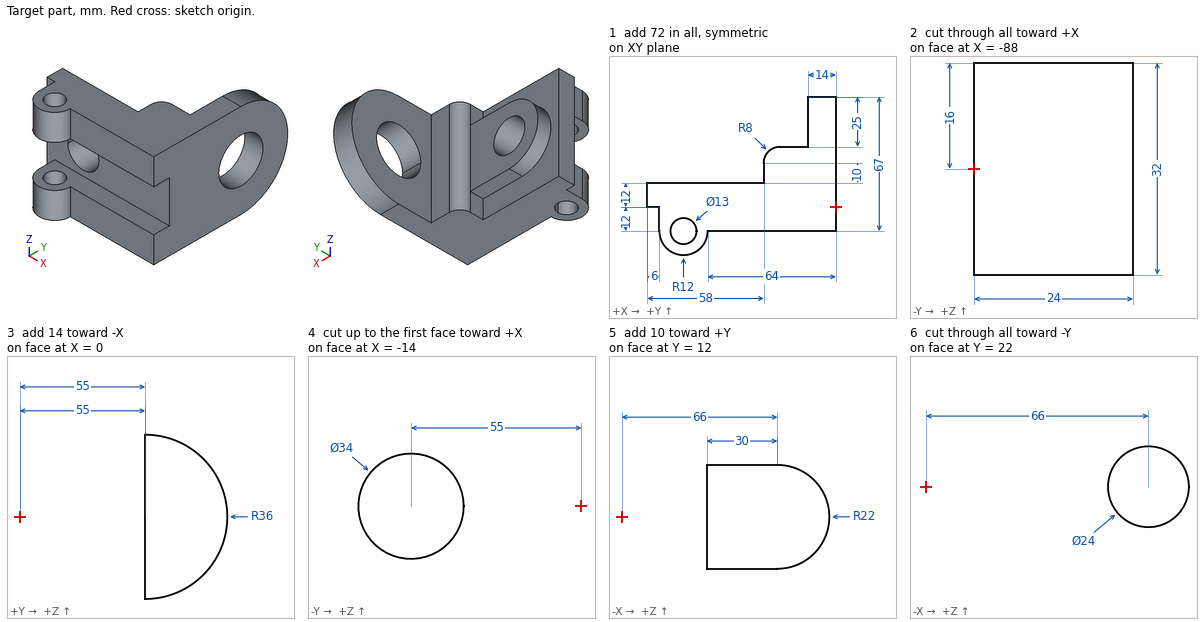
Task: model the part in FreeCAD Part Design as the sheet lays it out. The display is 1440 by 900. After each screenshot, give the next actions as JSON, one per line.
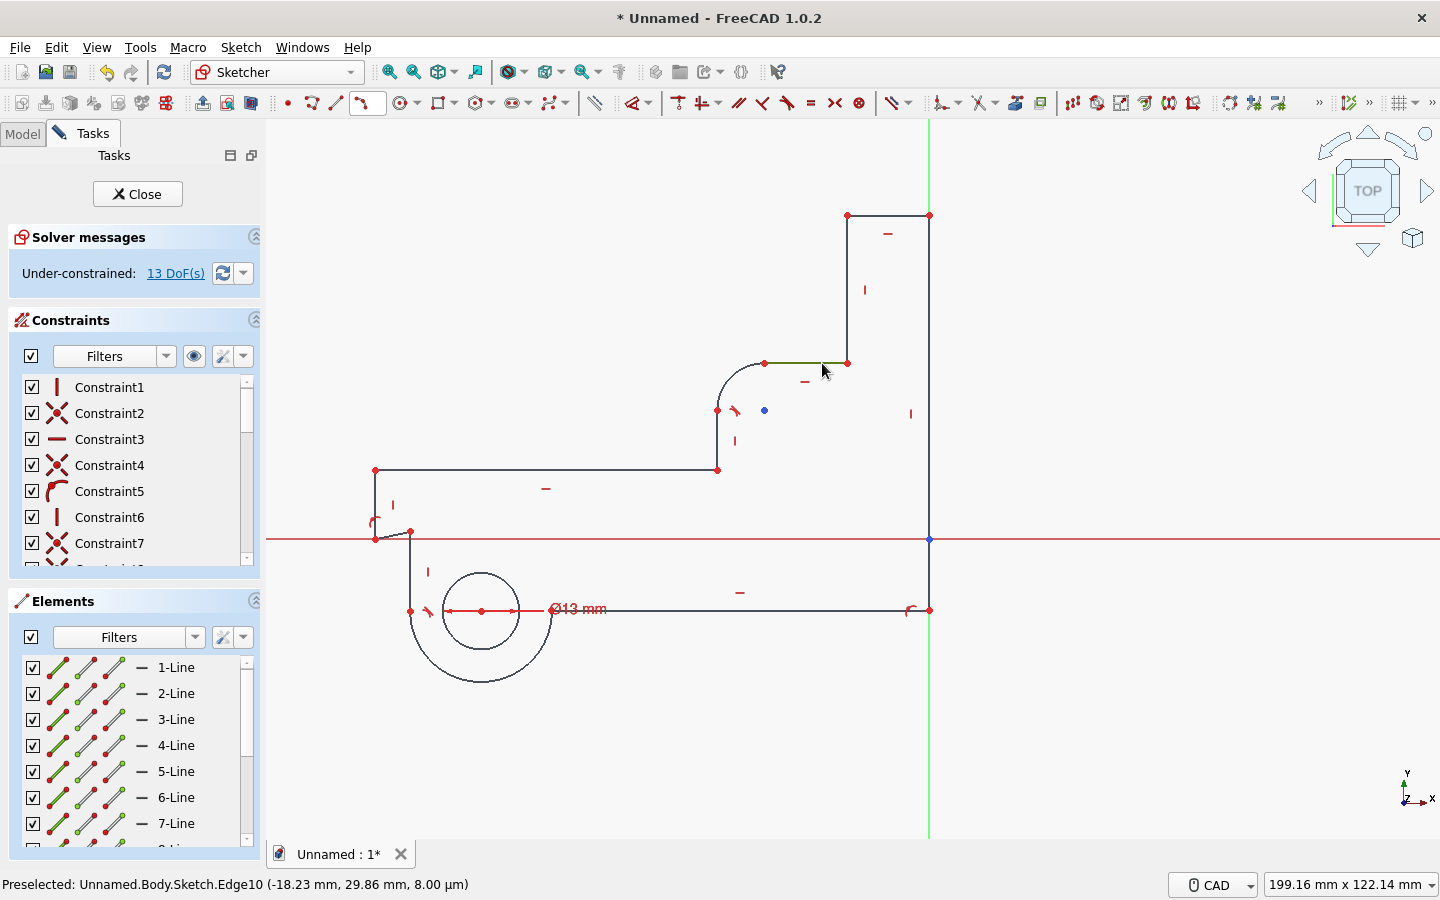
{"action": "left_click", "coordinate": [743, 368]}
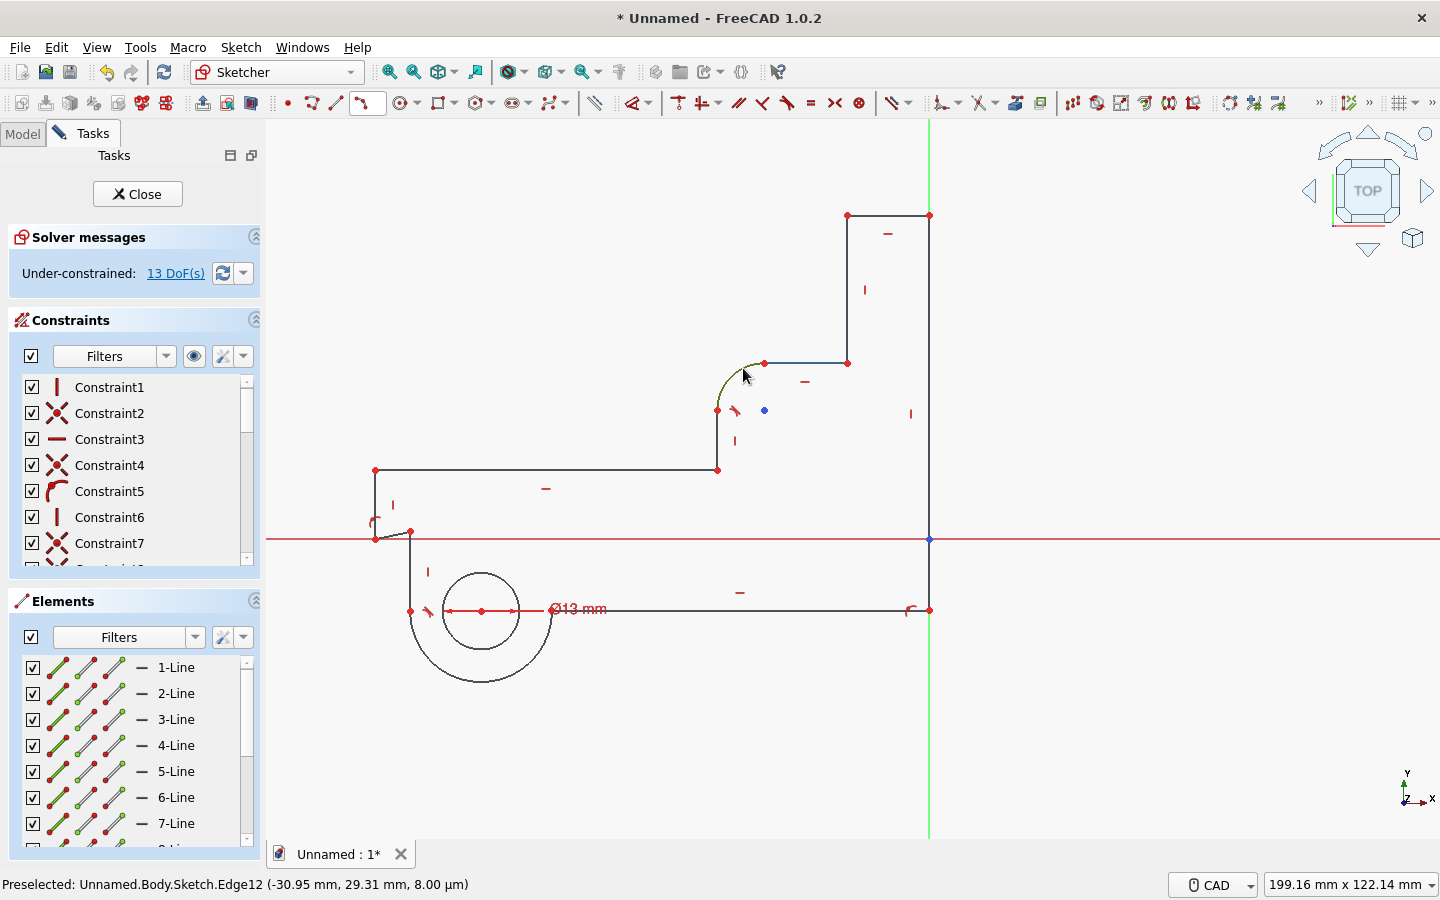
{"action": "left_click", "coordinate": [788, 104]}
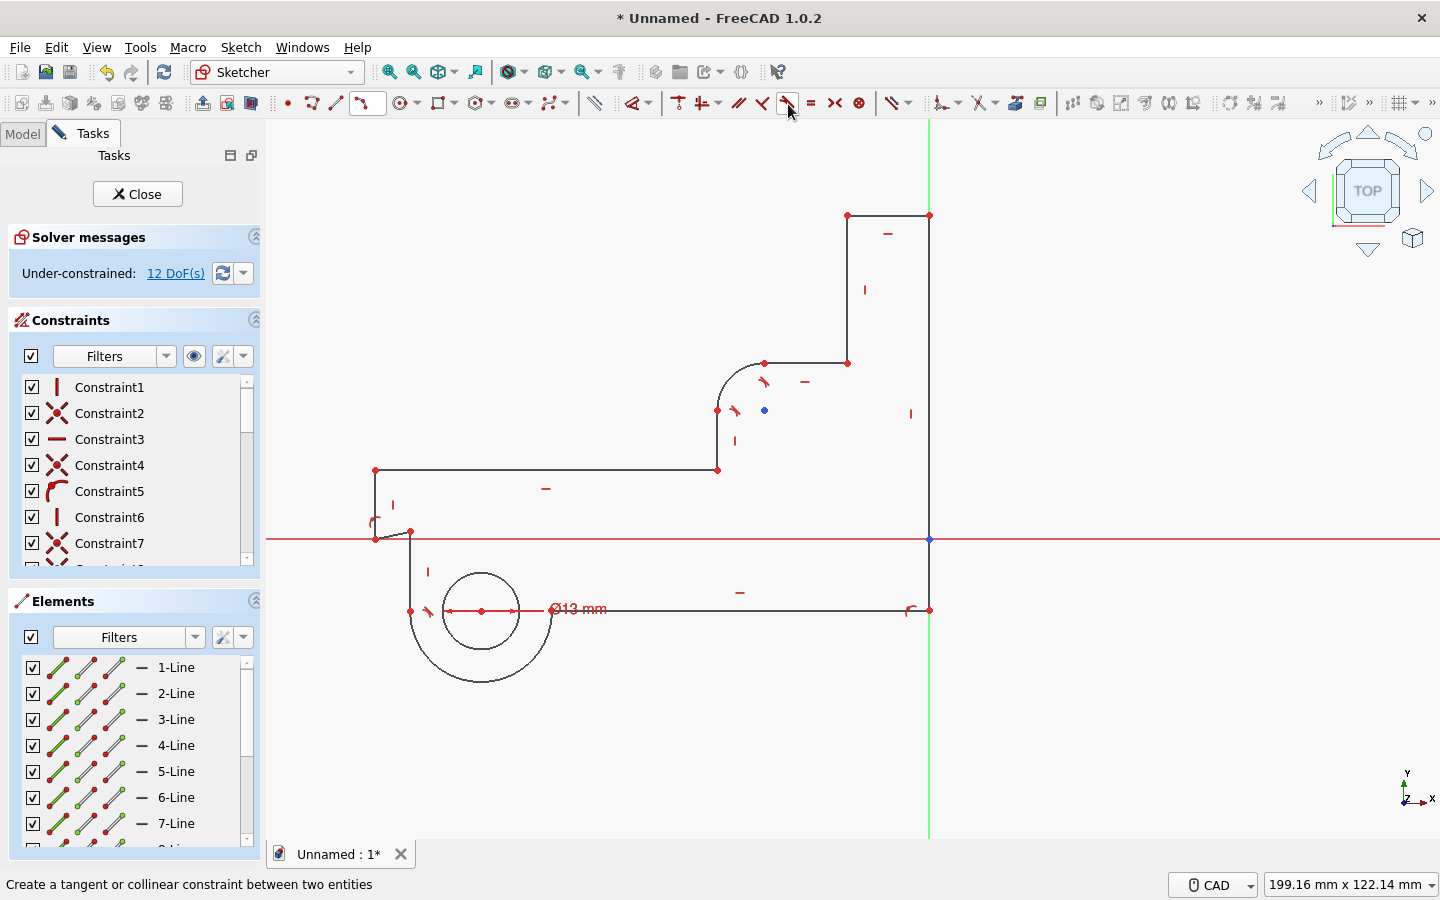
{"action": "scroll", "coordinate": [386, 537], "scroll_direction": "up", "scroll_amount": 2}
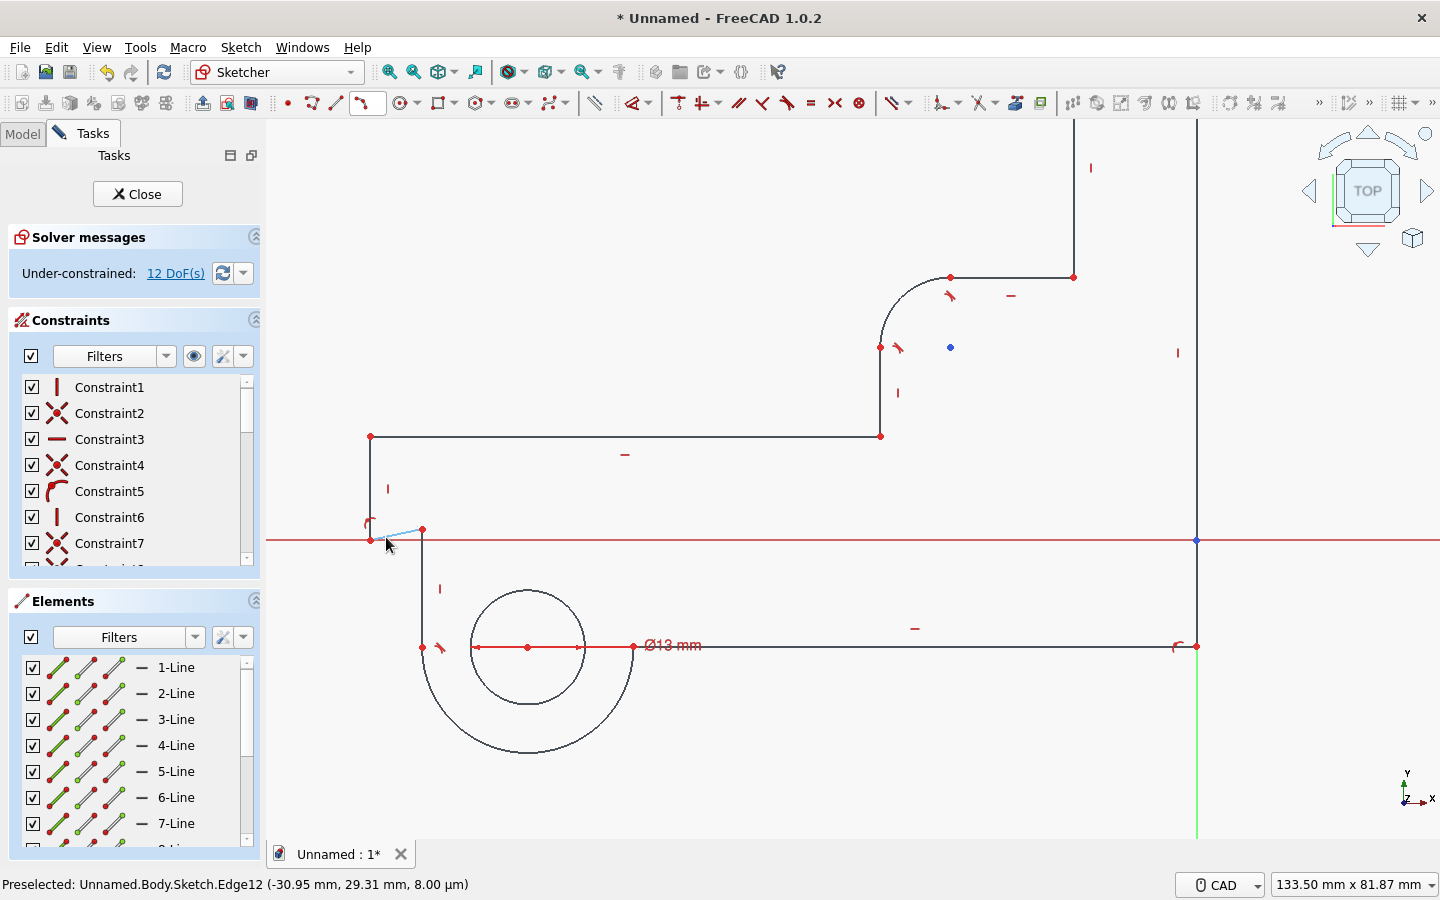
{"action": "left_click", "coordinate": [386, 537]}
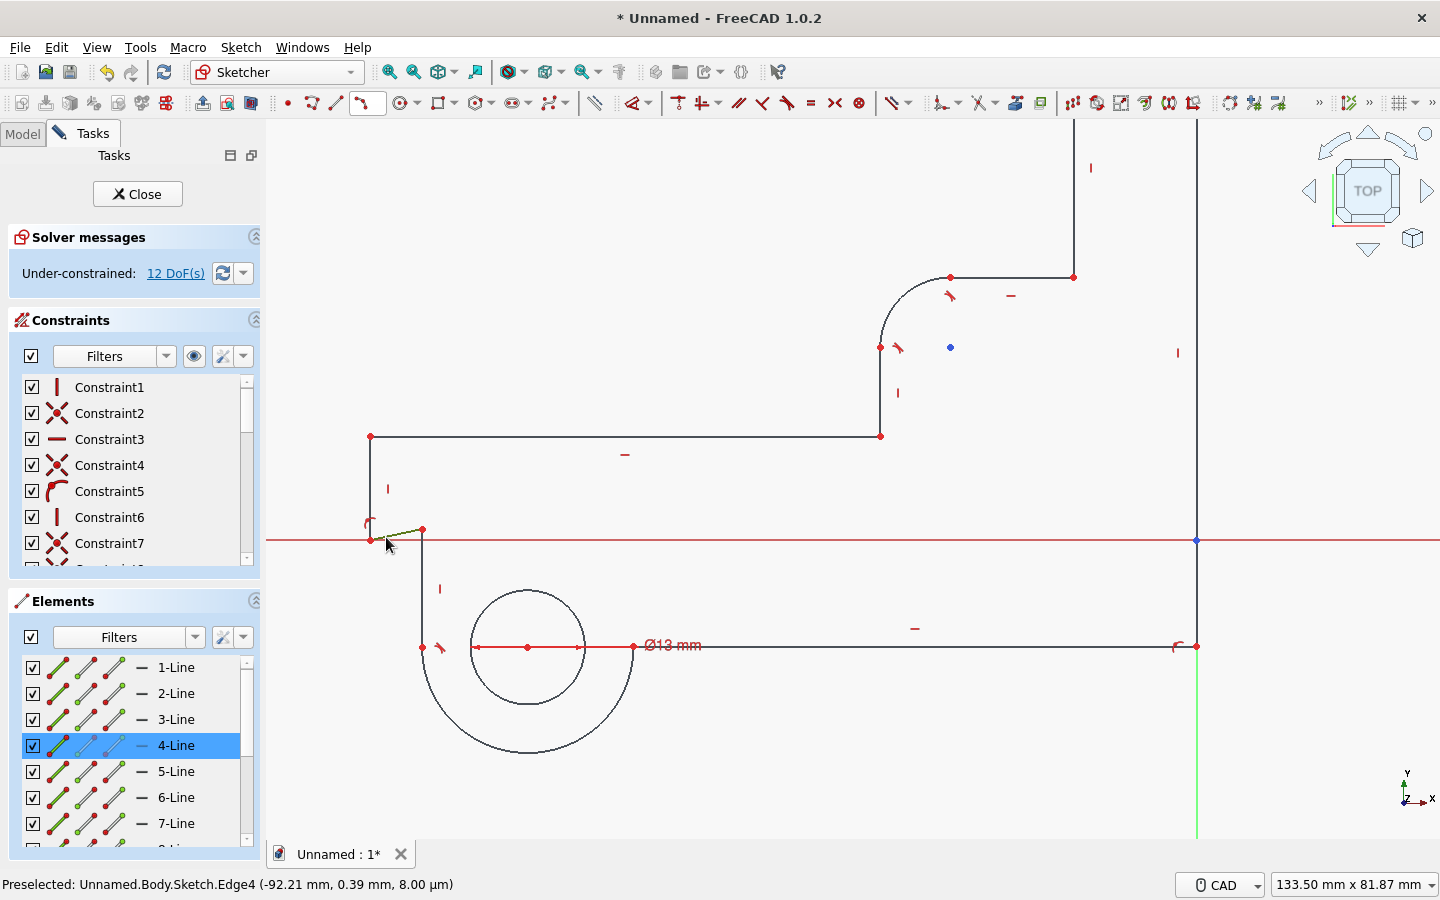
{"action": "key", "text": "h"}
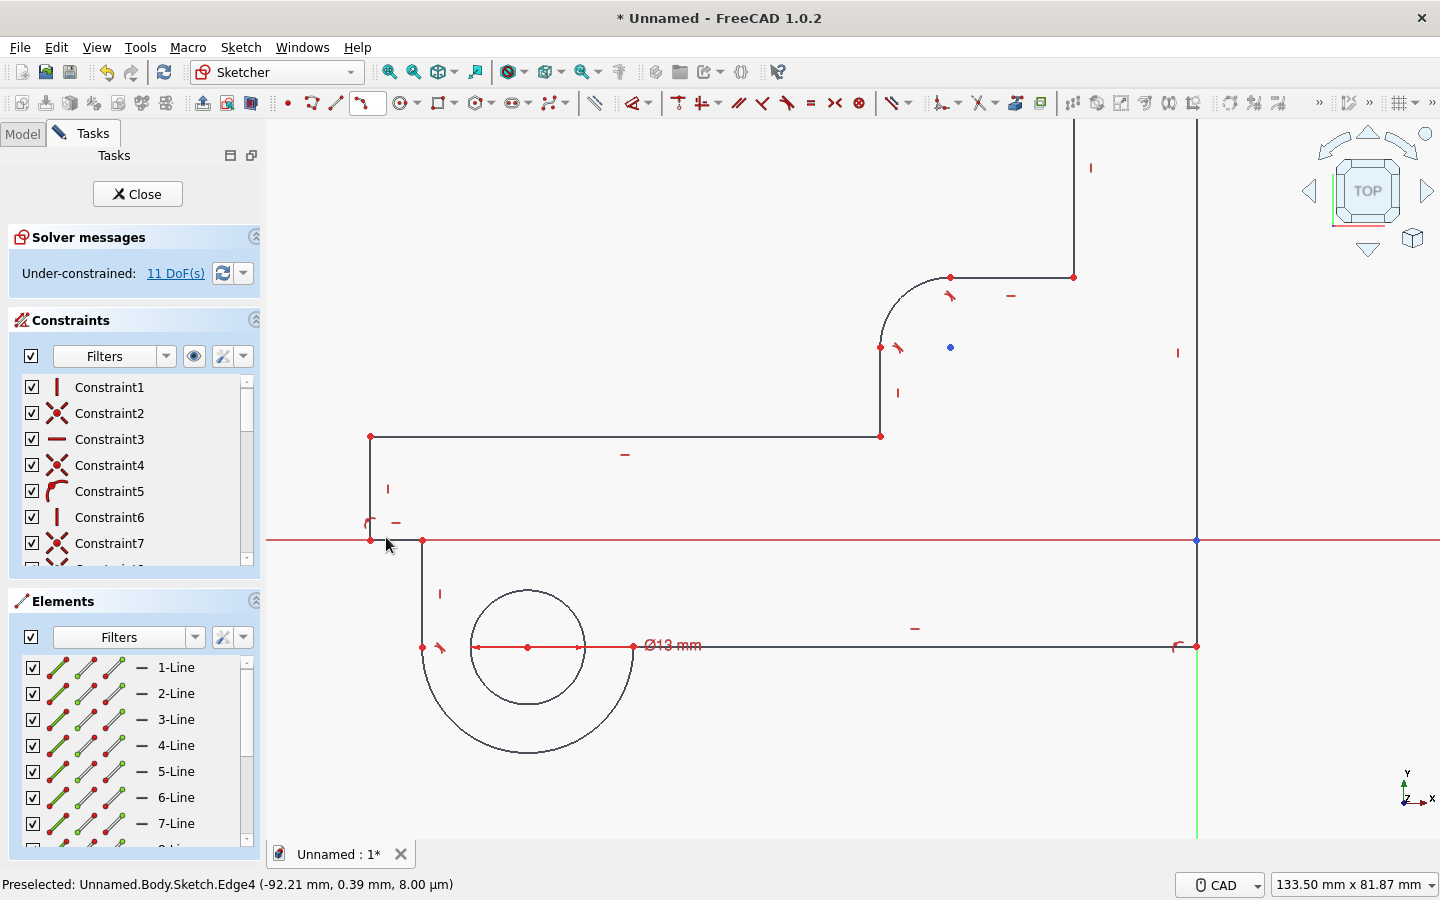
{"action": "left_click", "coordinate": [632, 104]}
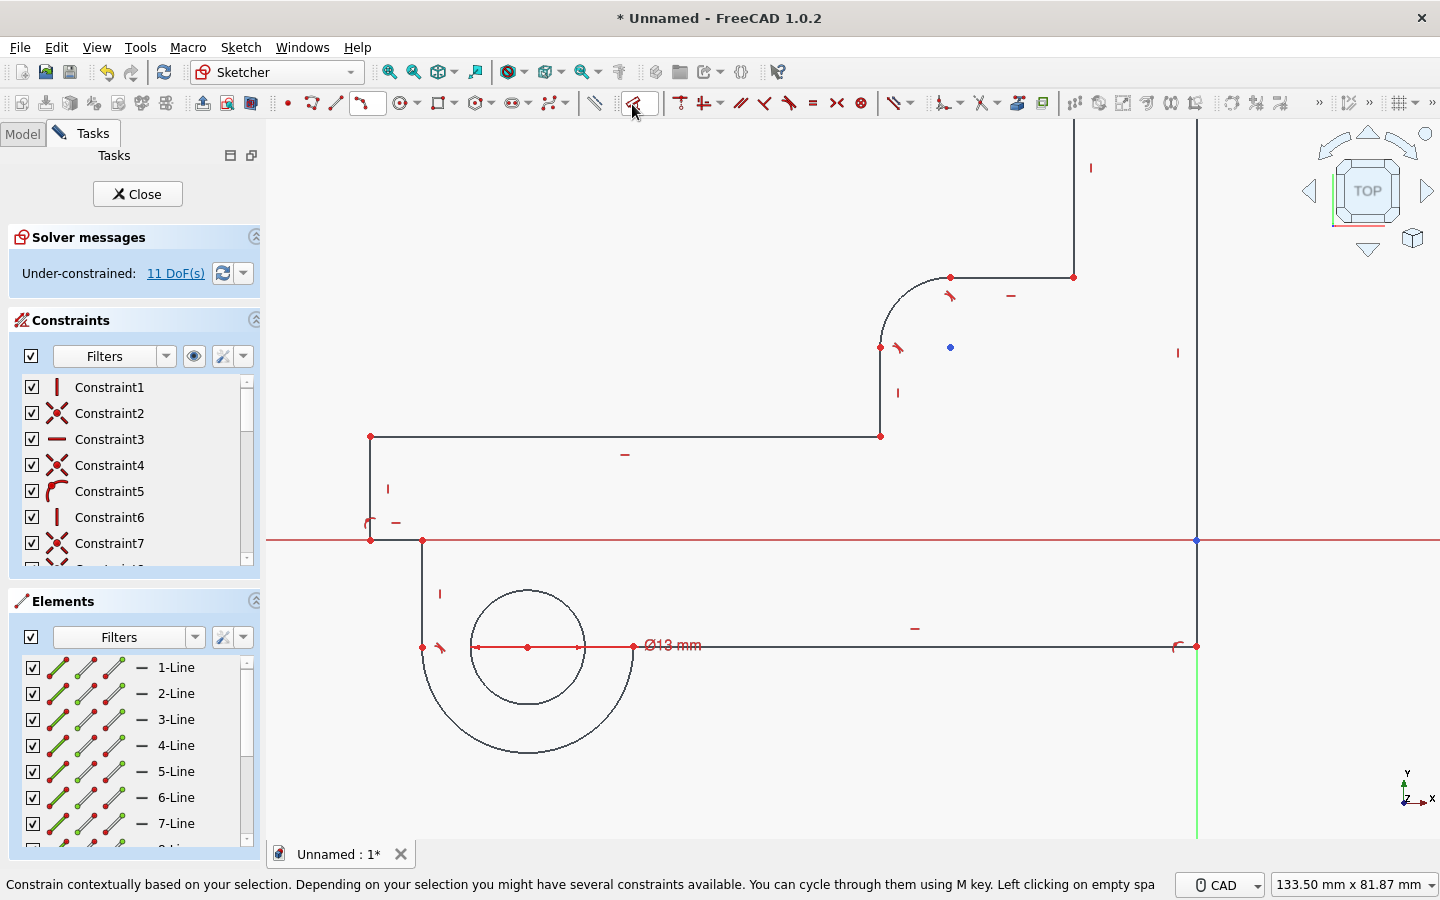
{"action": "left_click", "coordinate": [466, 733]}
{"action": "left_click", "coordinate": [447, 759]}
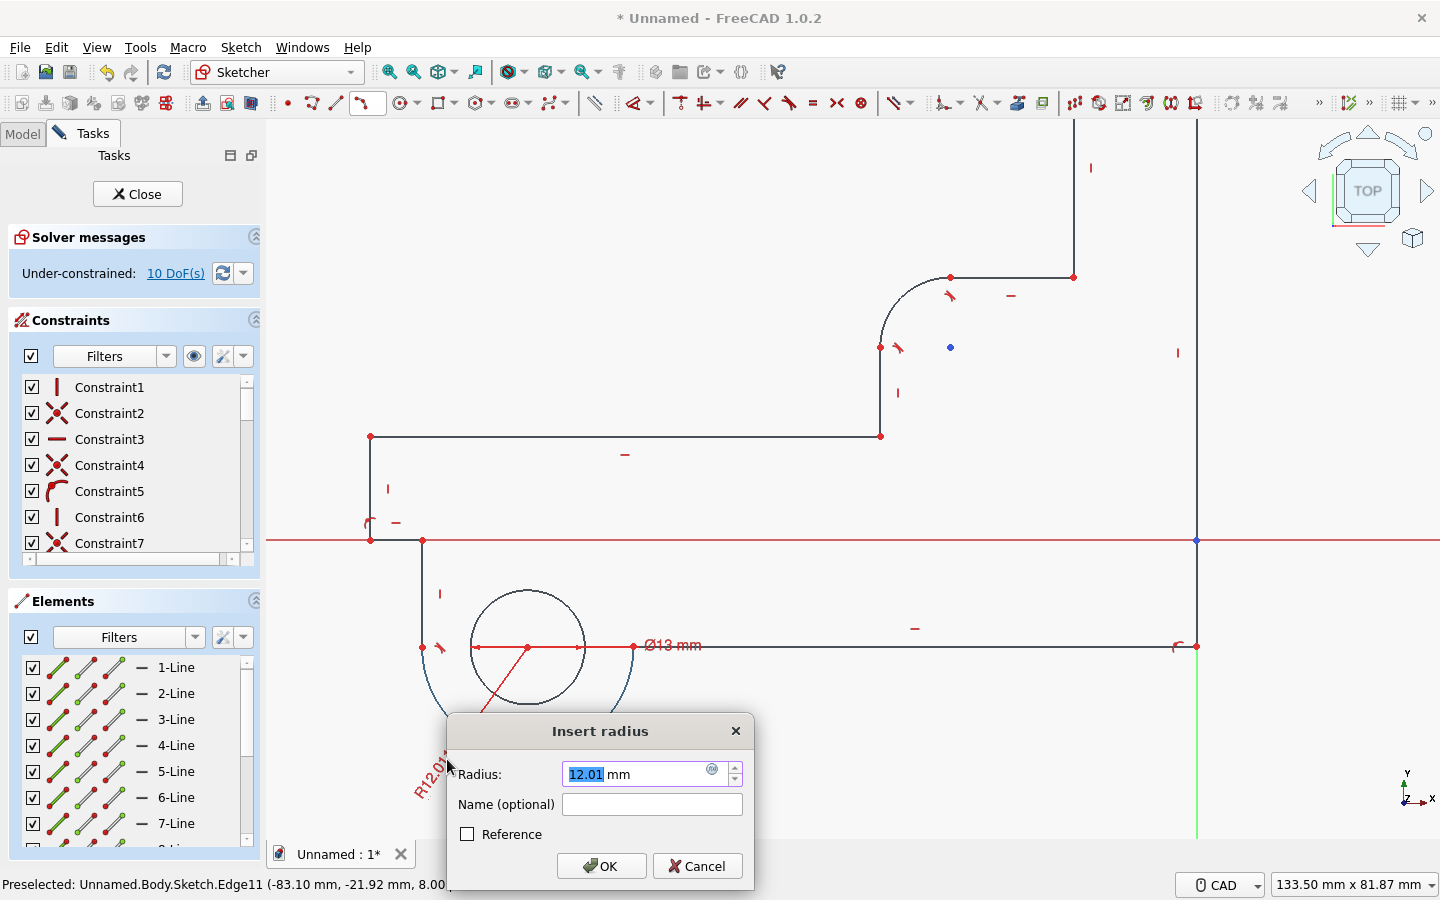
{"action": "type", "text": "12"}
{"action": "key", "text": "Return"}